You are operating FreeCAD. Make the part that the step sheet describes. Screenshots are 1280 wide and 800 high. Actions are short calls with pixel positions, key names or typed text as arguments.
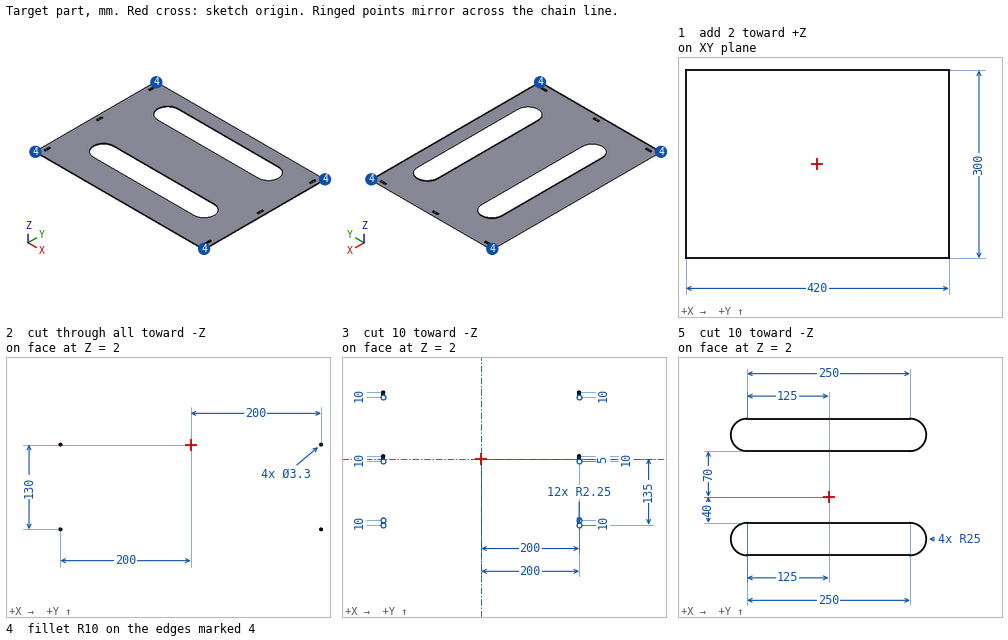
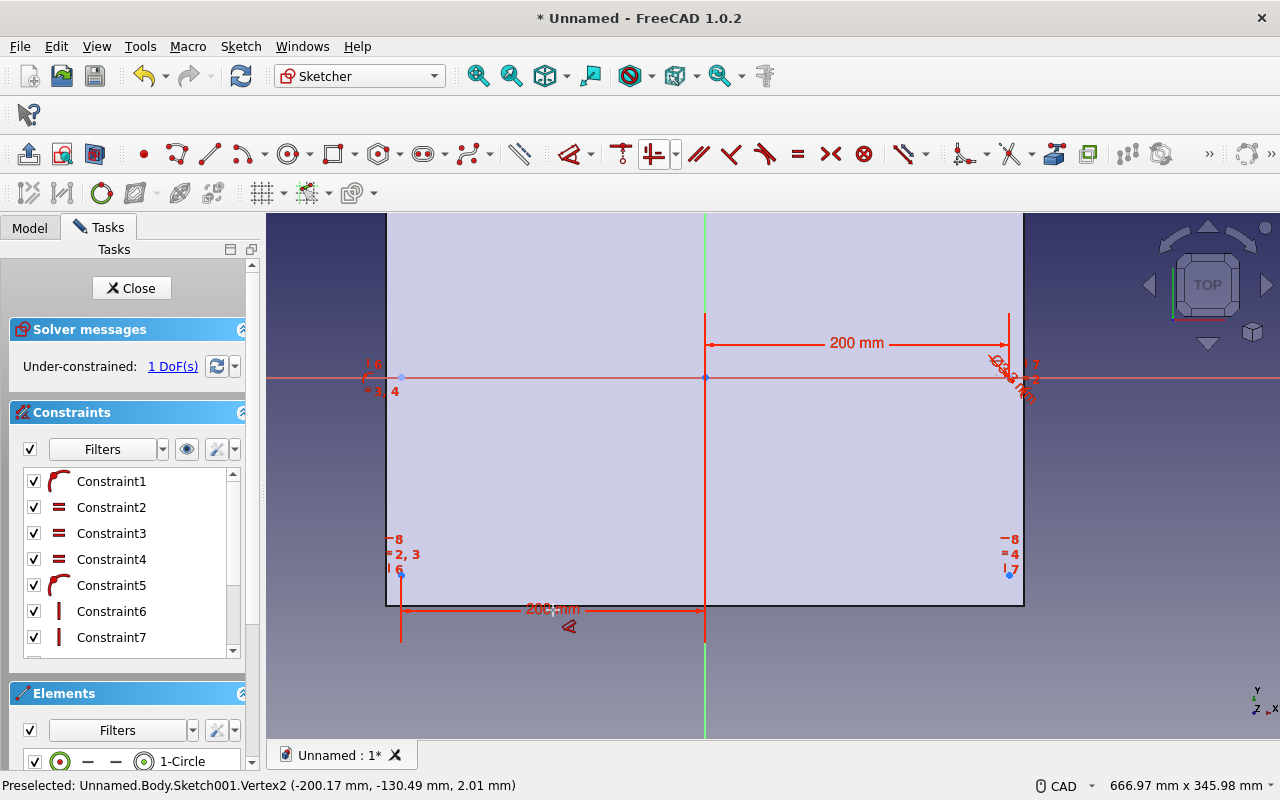
click(401, 576)
click(367, 477)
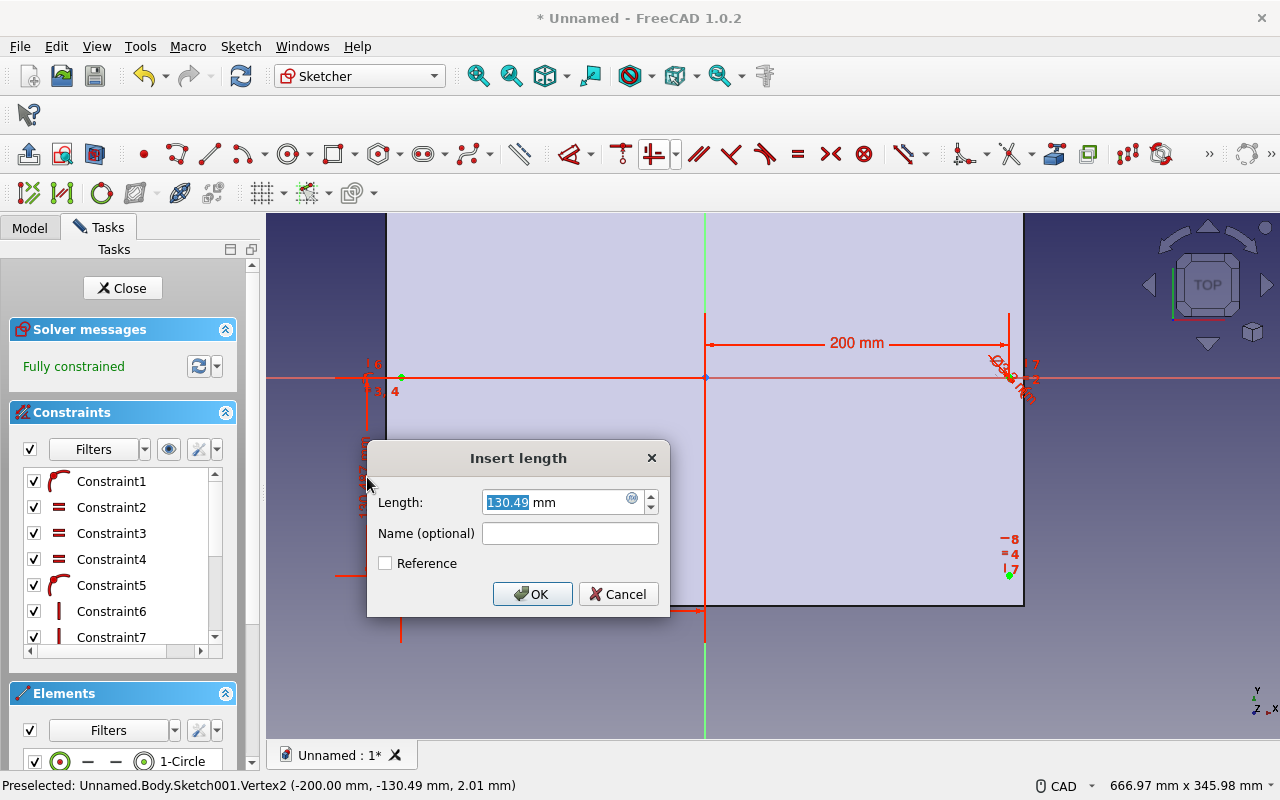
text(130)
key(Return)
key(Escape)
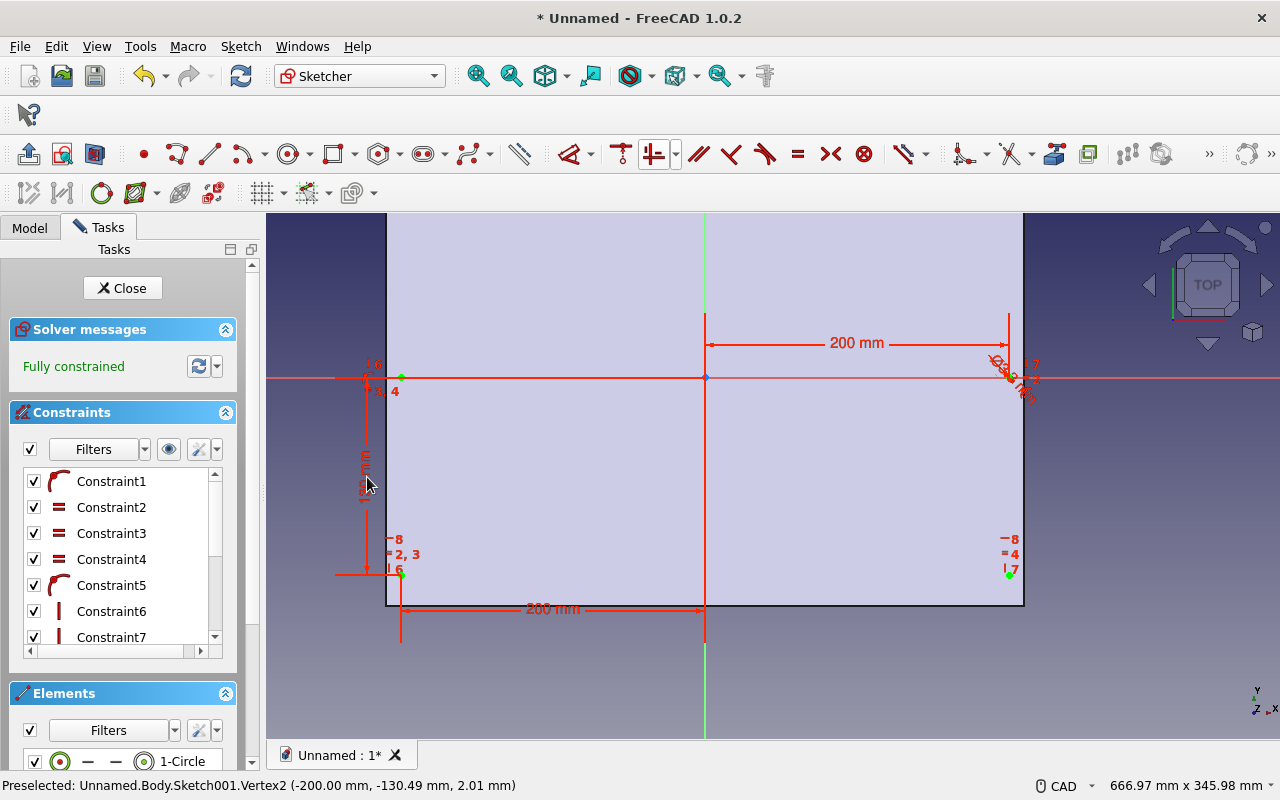
click(123, 288)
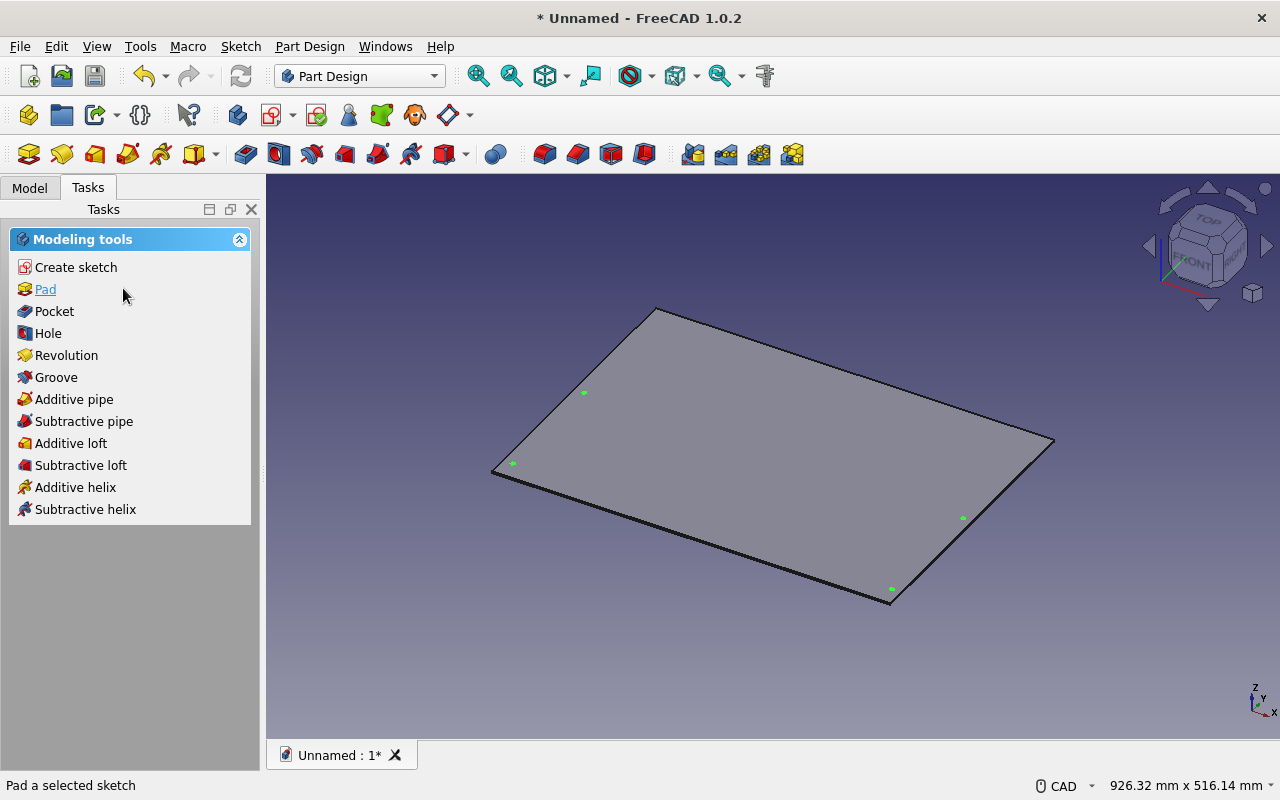
click(246, 154)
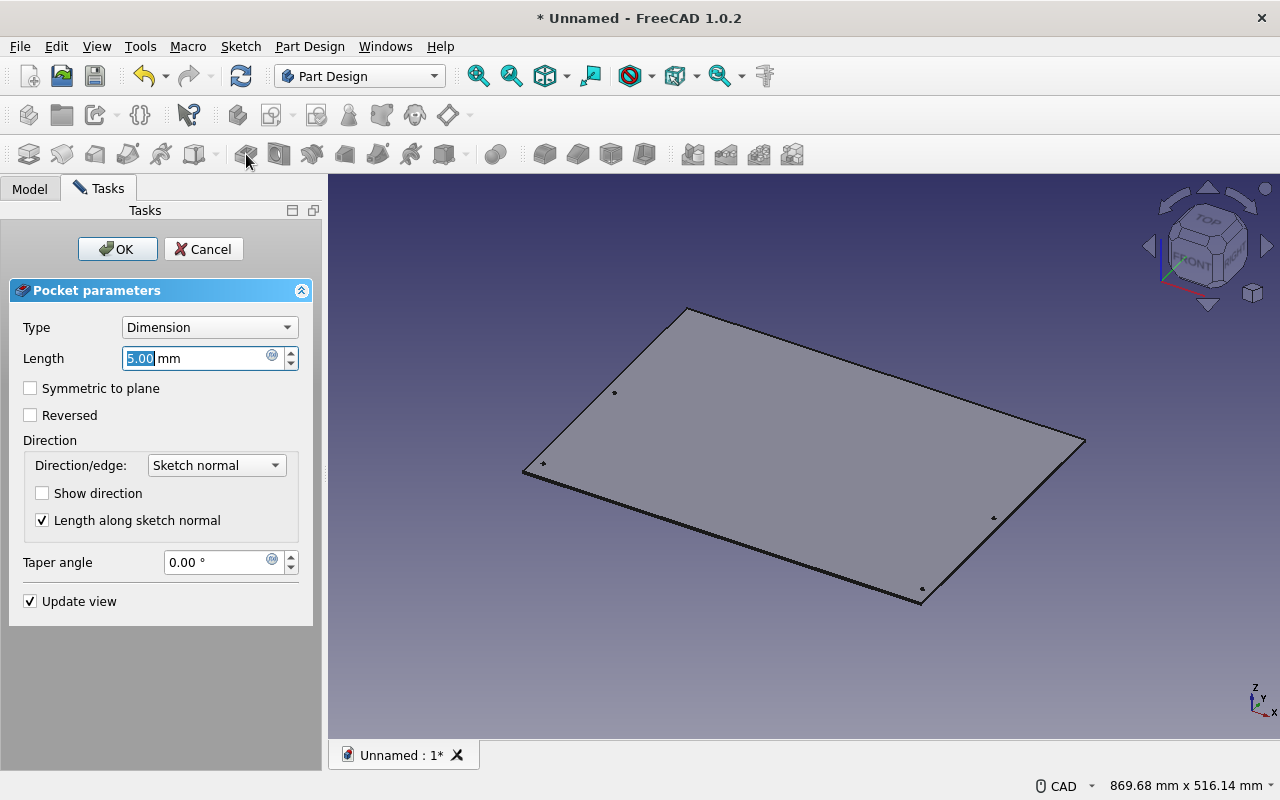
click(210, 328)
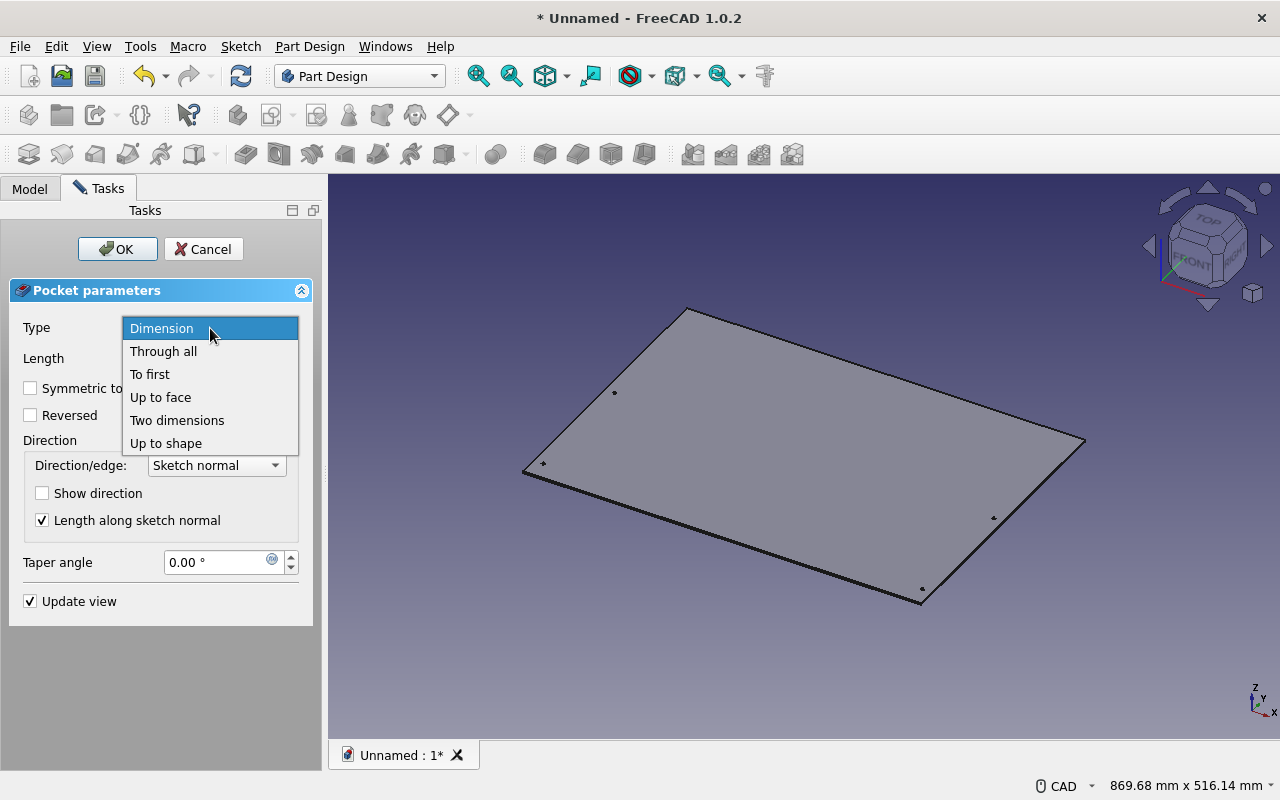
click(208, 352)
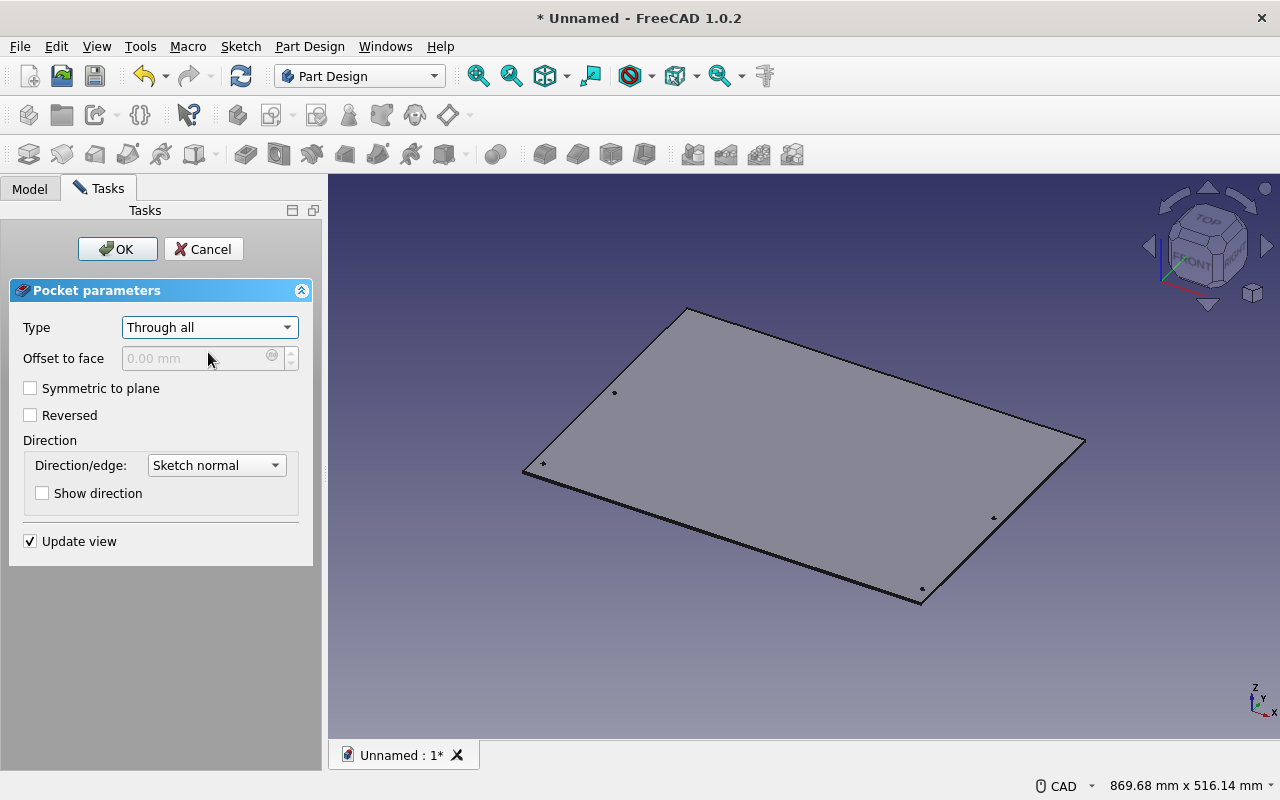
click(118, 249)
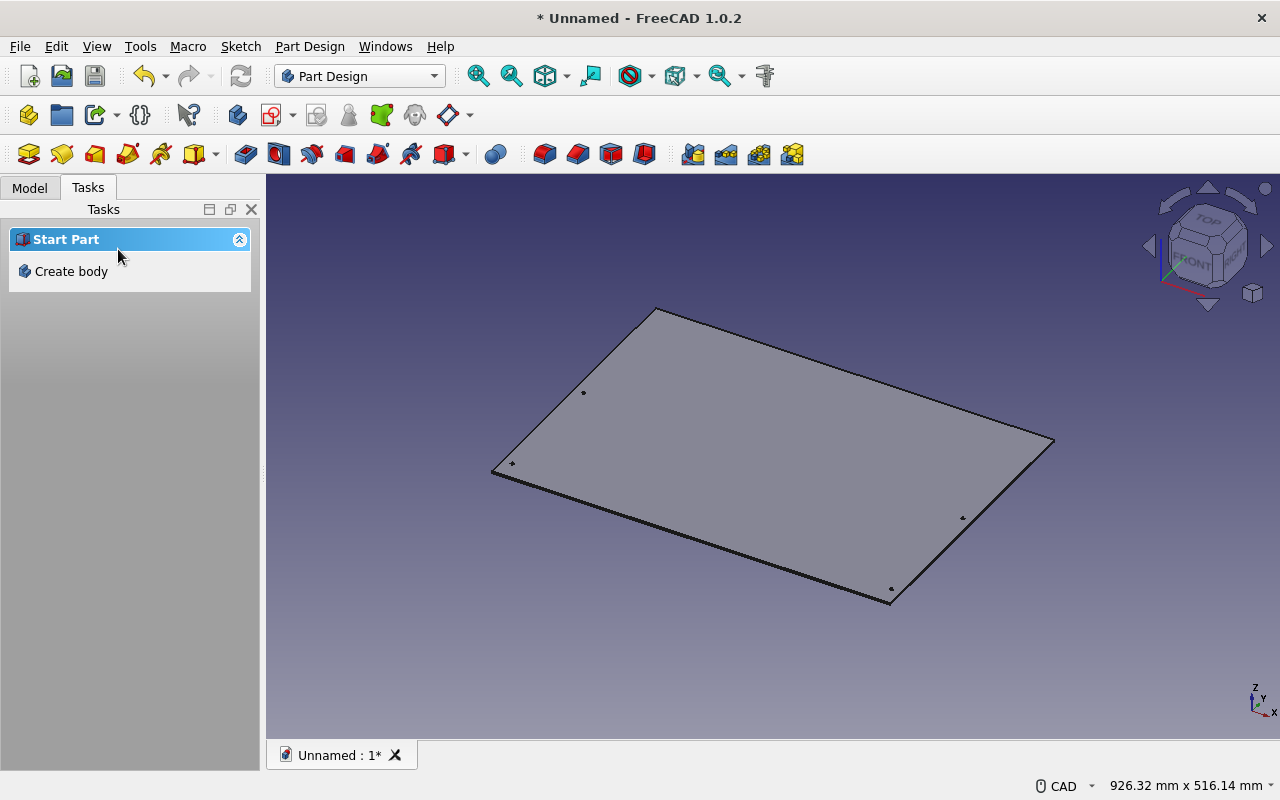
click(773, 455)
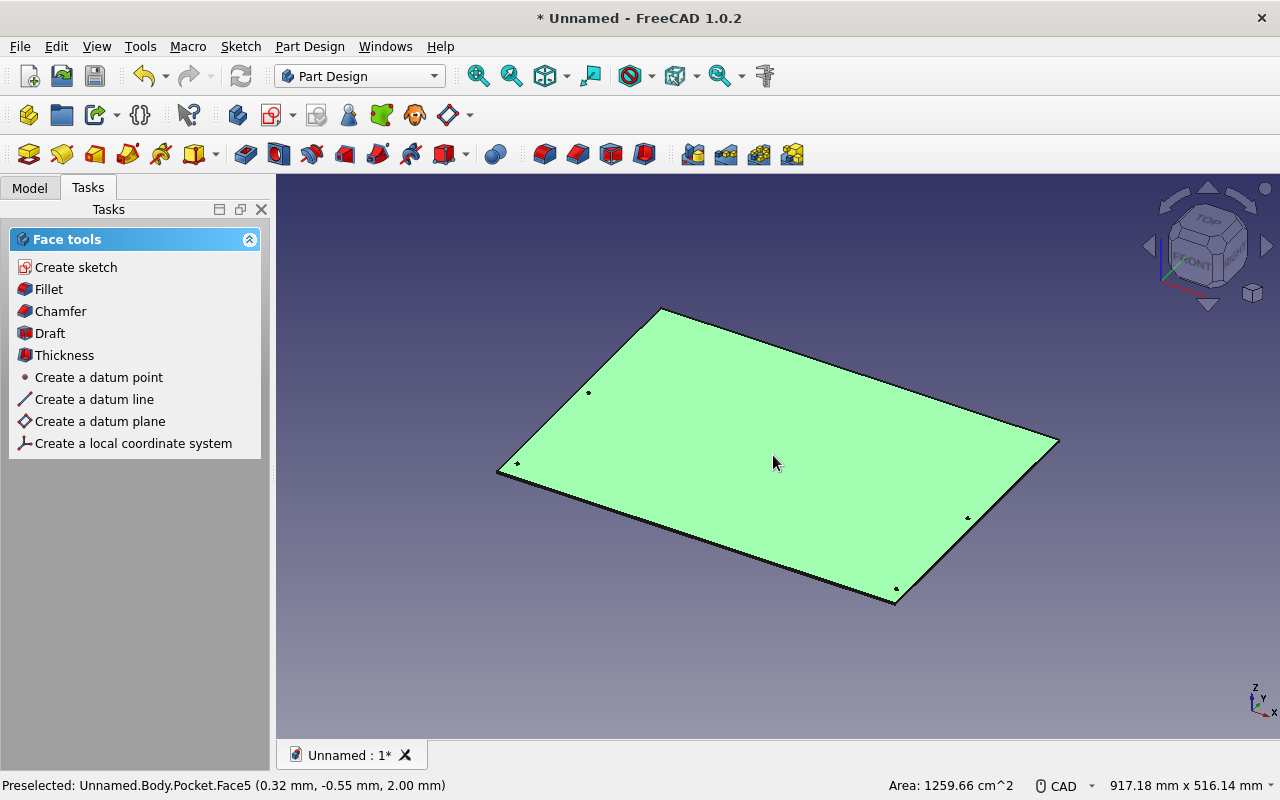
click(270, 116)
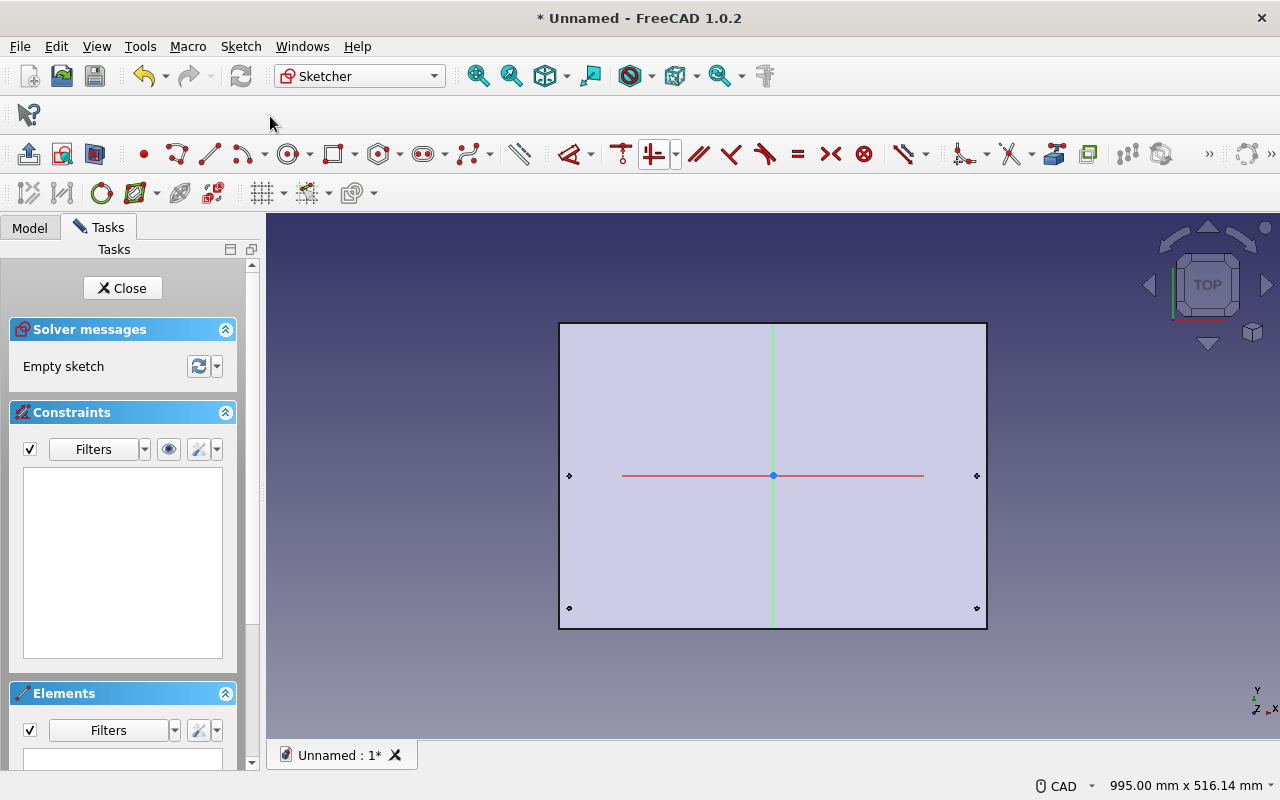
click(422, 154)